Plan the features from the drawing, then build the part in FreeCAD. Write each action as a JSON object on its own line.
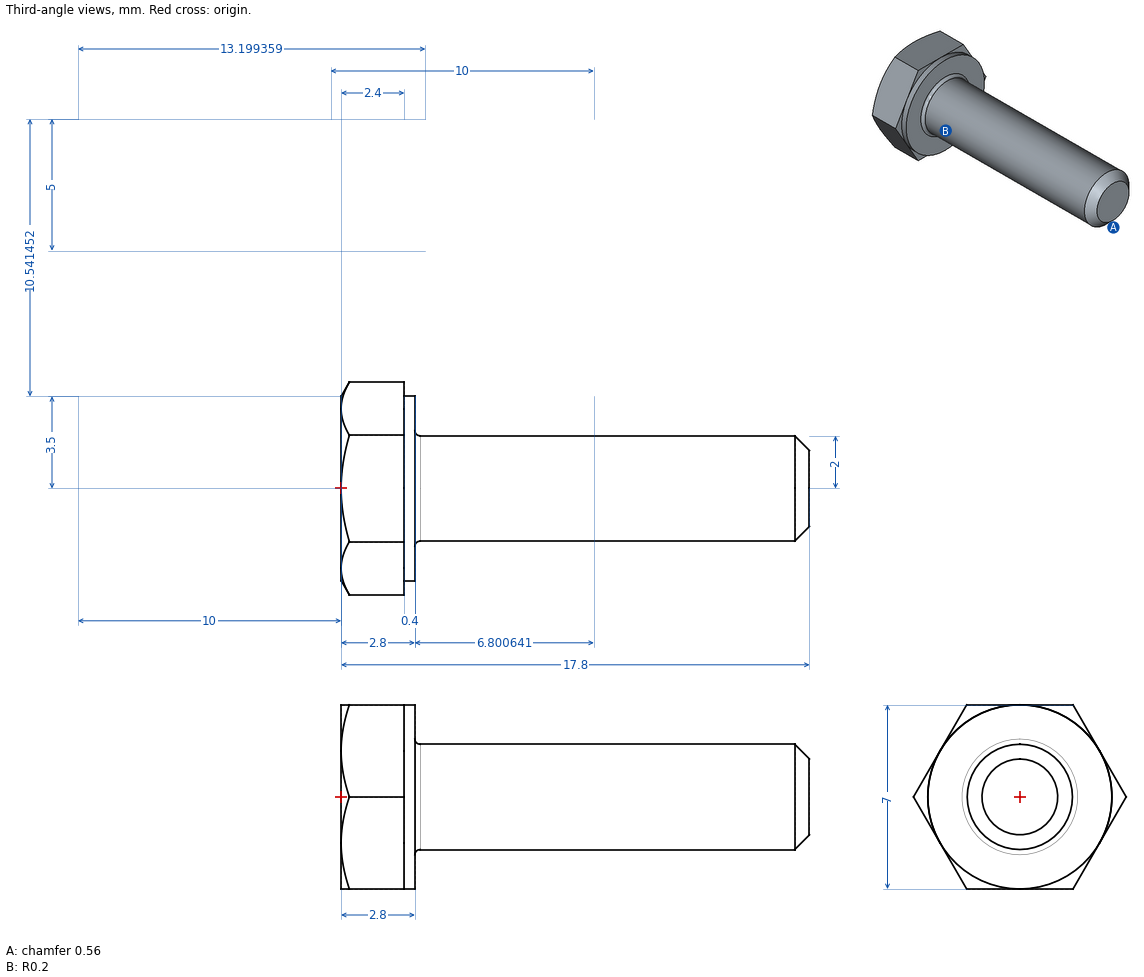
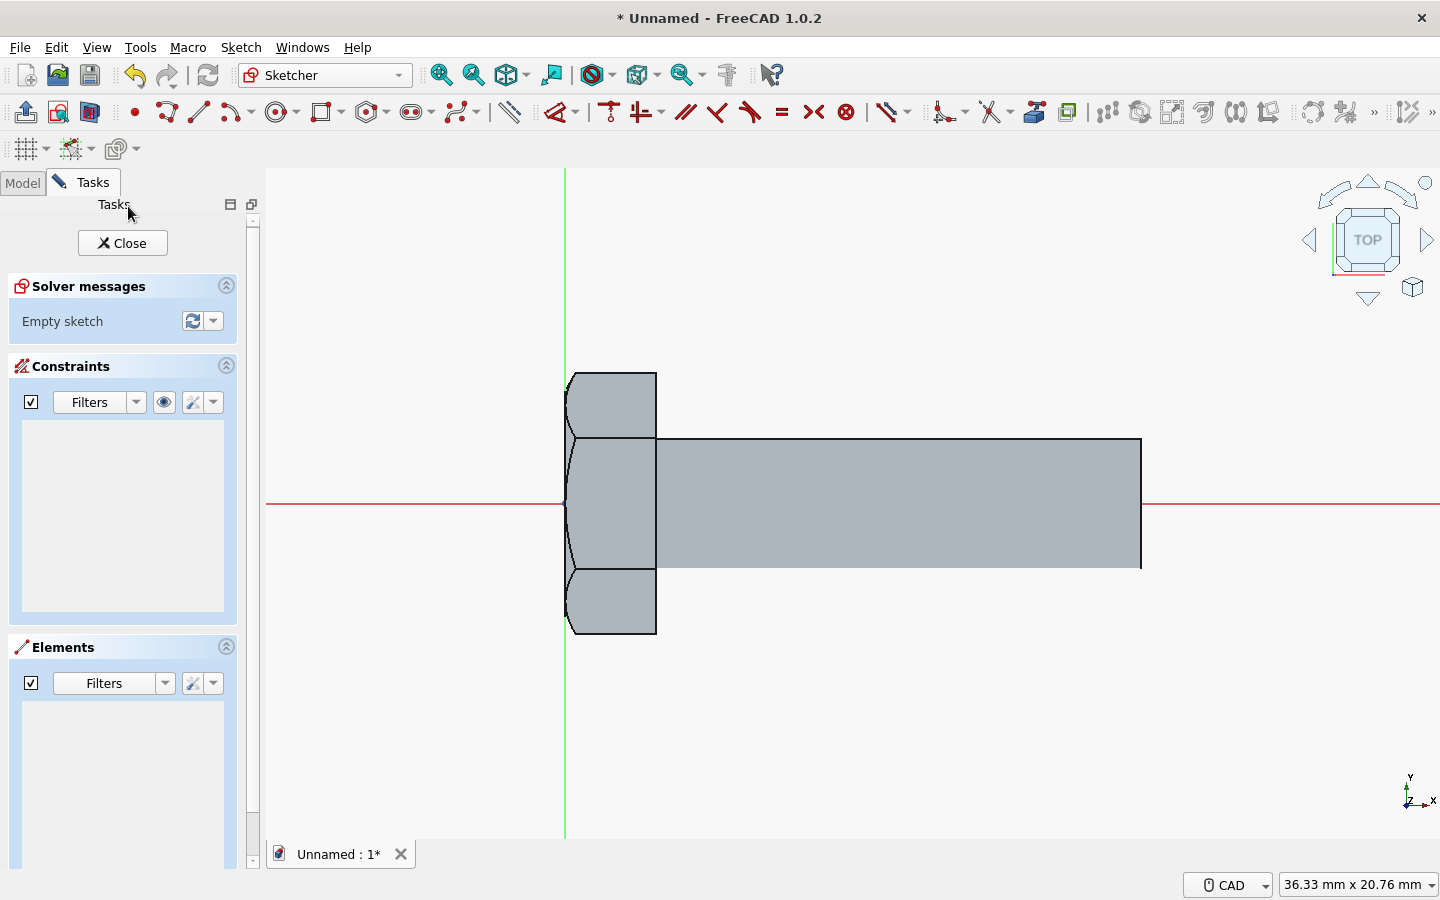
{"action": "left_click", "coordinate": [90, 112]}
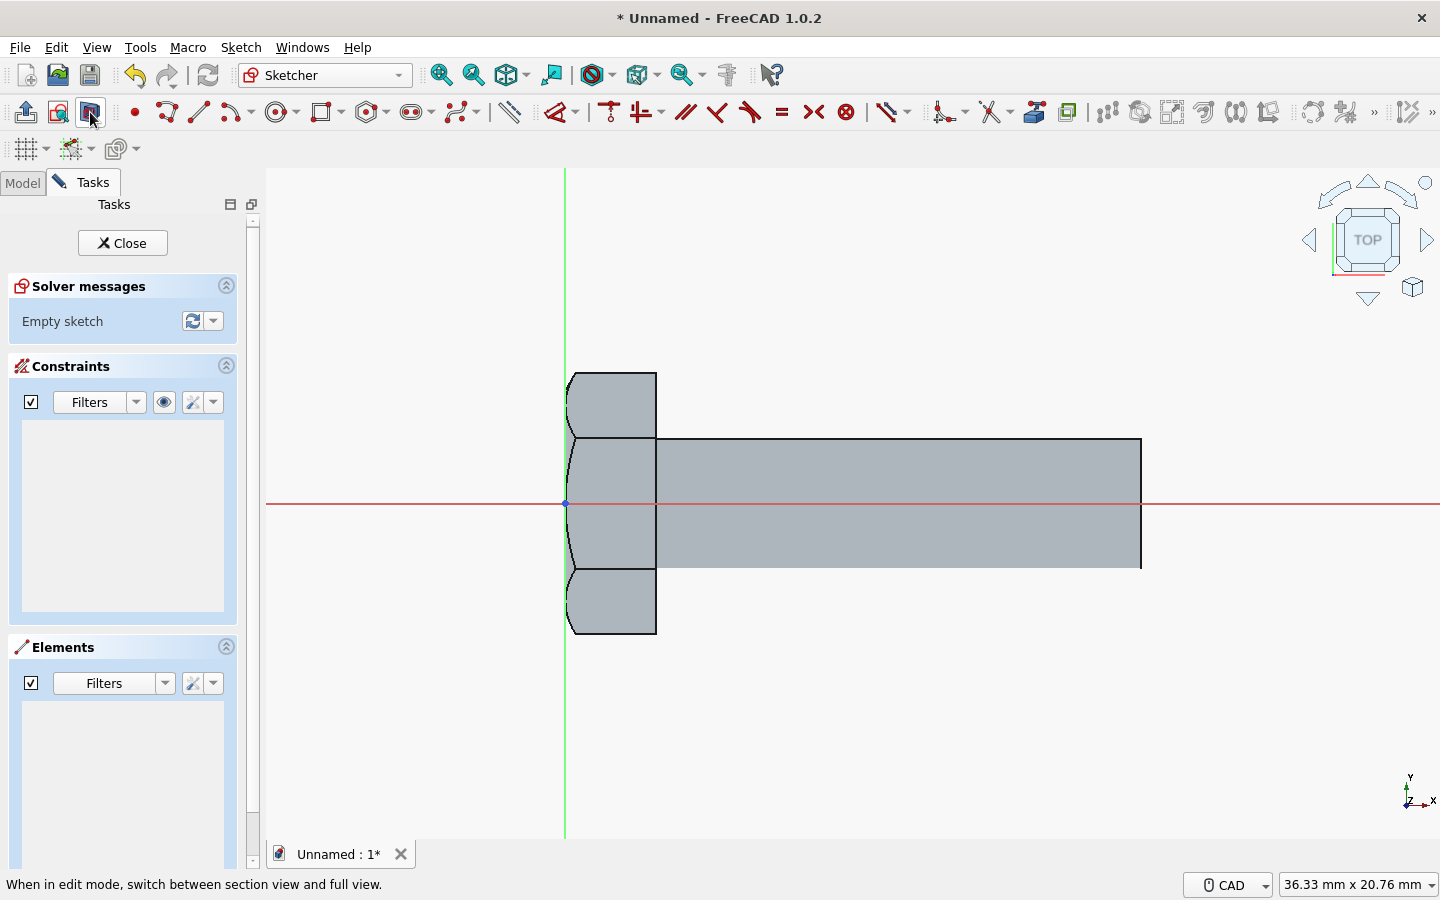
{"action": "scroll", "coordinate": [928, 811], "scroll_direction": "down", "scroll_amount": 2}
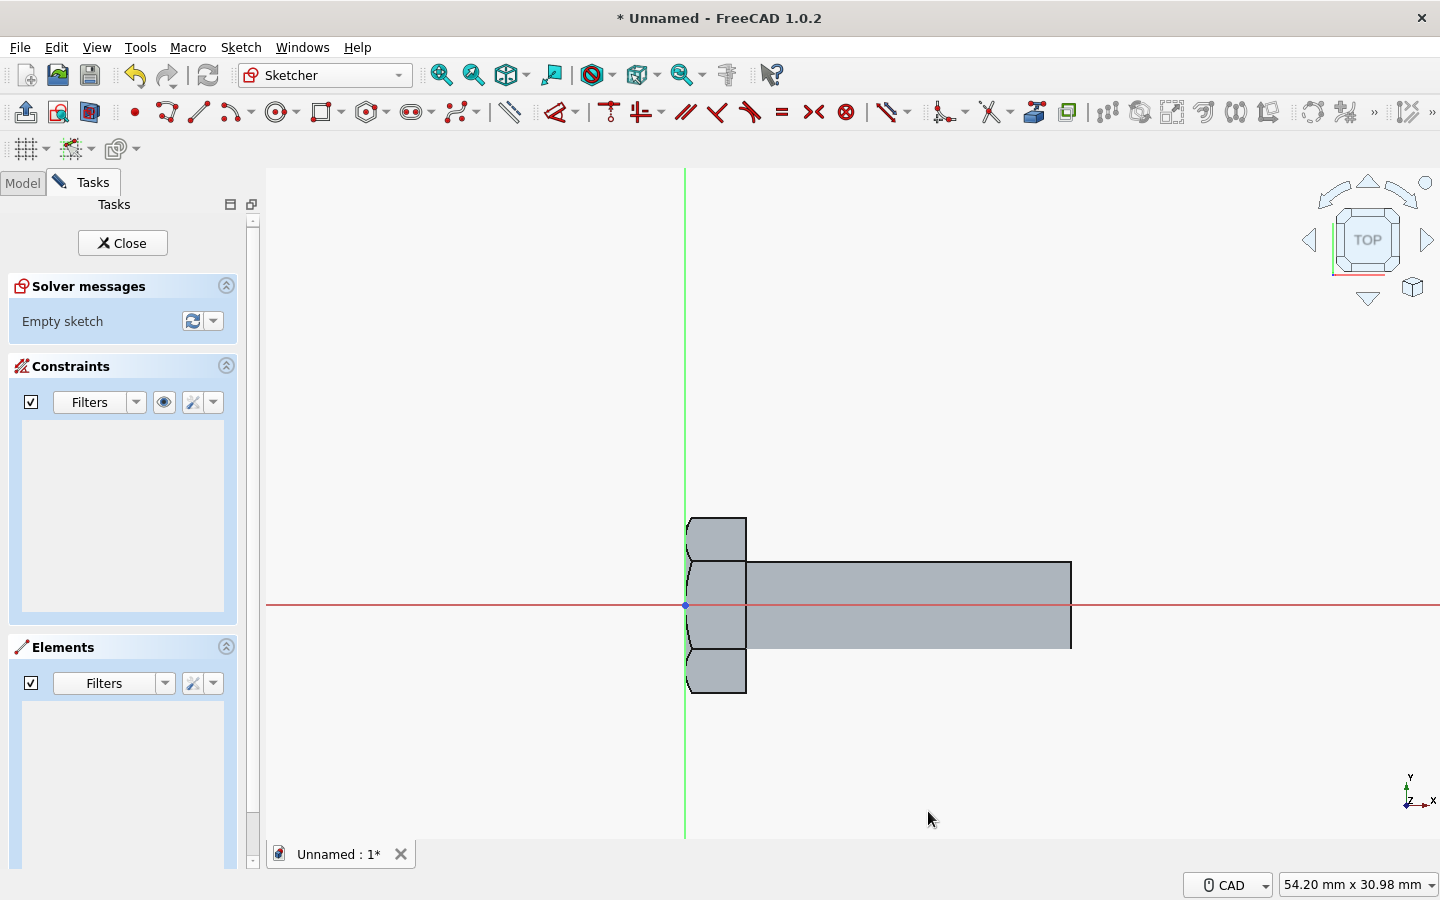
{"action": "scroll", "coordinate": [785, 351], "scroll_direction": "up", "scroll_amount": 2}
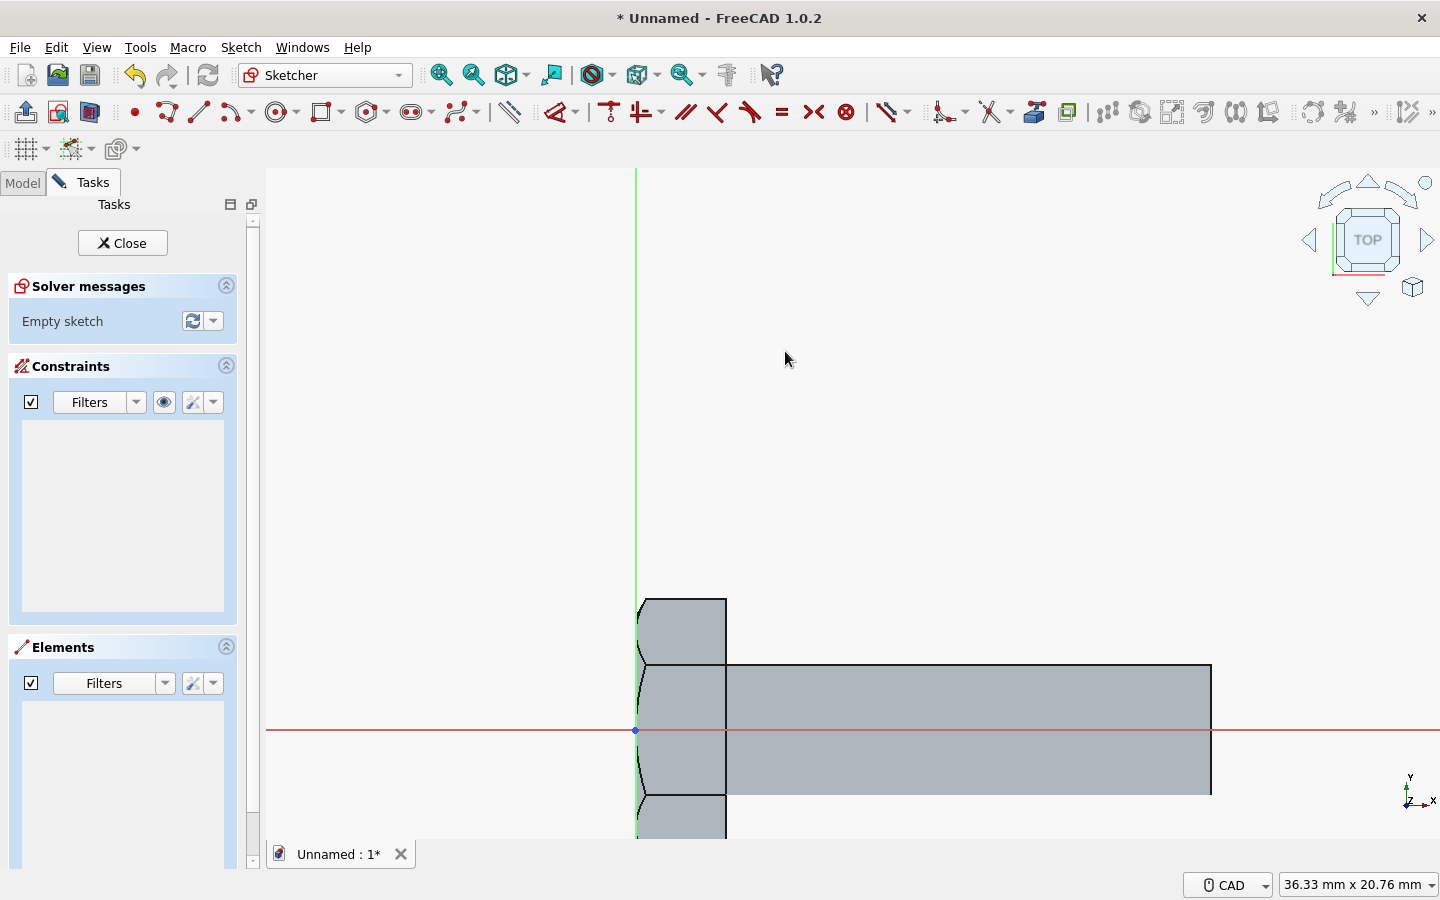
{"action": "key", "text": "g m"}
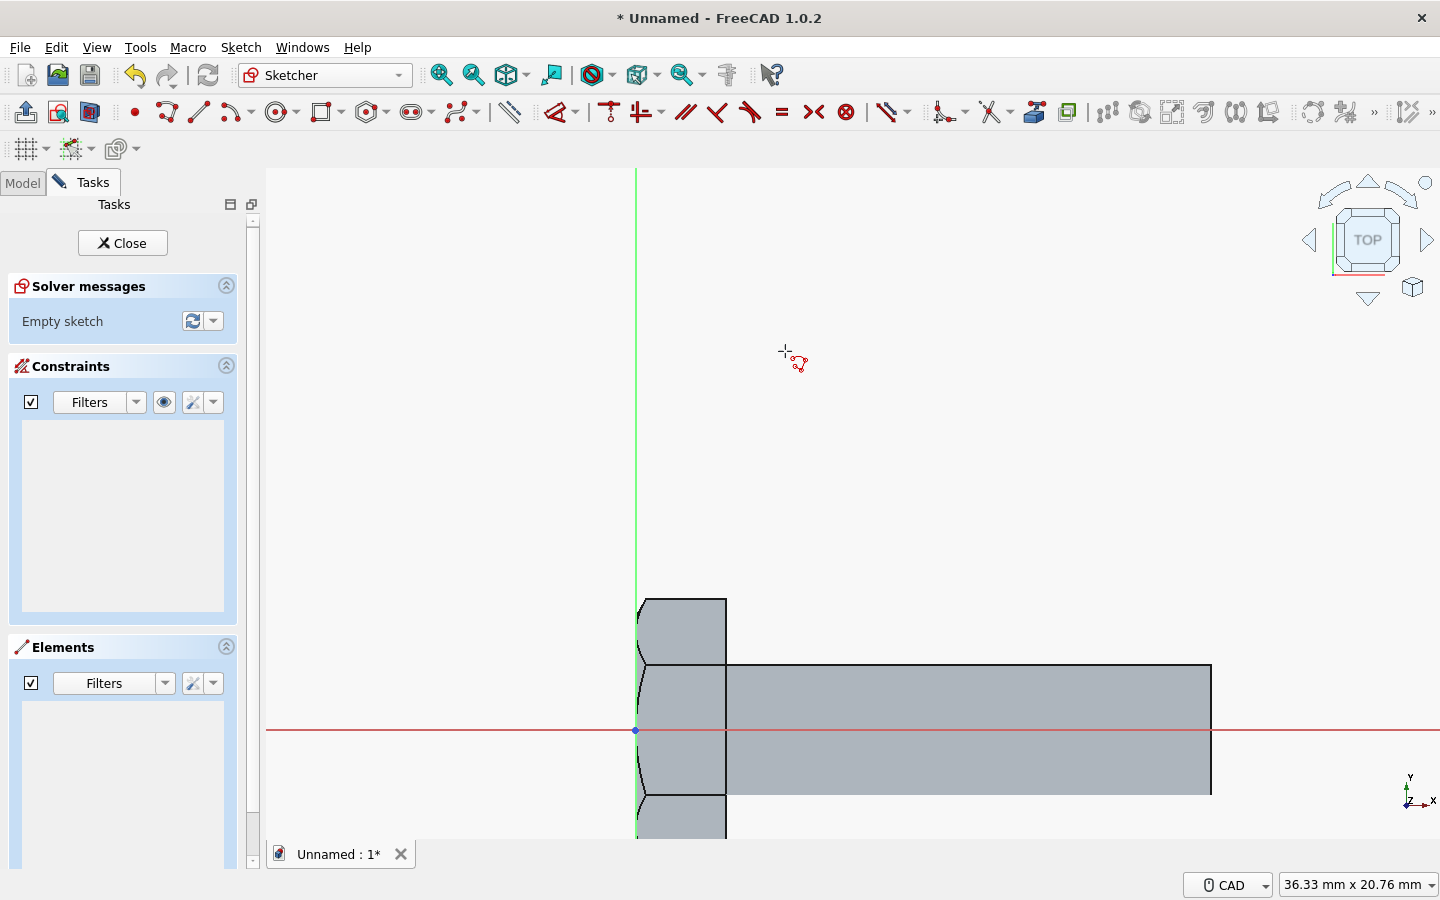
{"action": "left_click", "coordinate": [726, 617]}
{"action": "left_click", "coordinate": [946, 617]}
{"action": "left_click", "coordinate": [946, 276]}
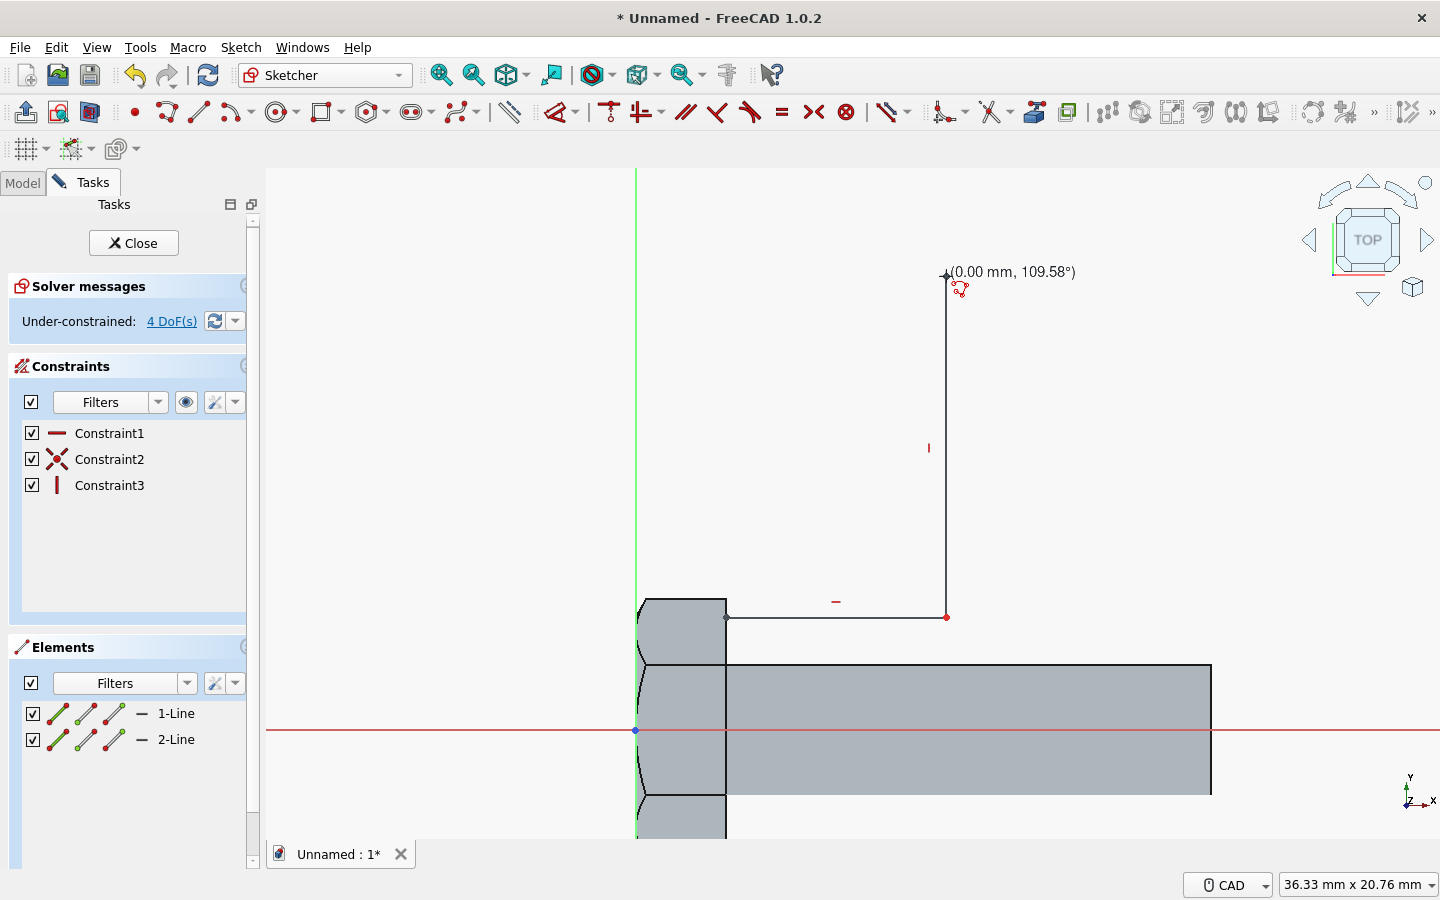
{"action": "scroll", "coordinate": [623, 276], "scroll_direction": "up", "scroll_amount": 2}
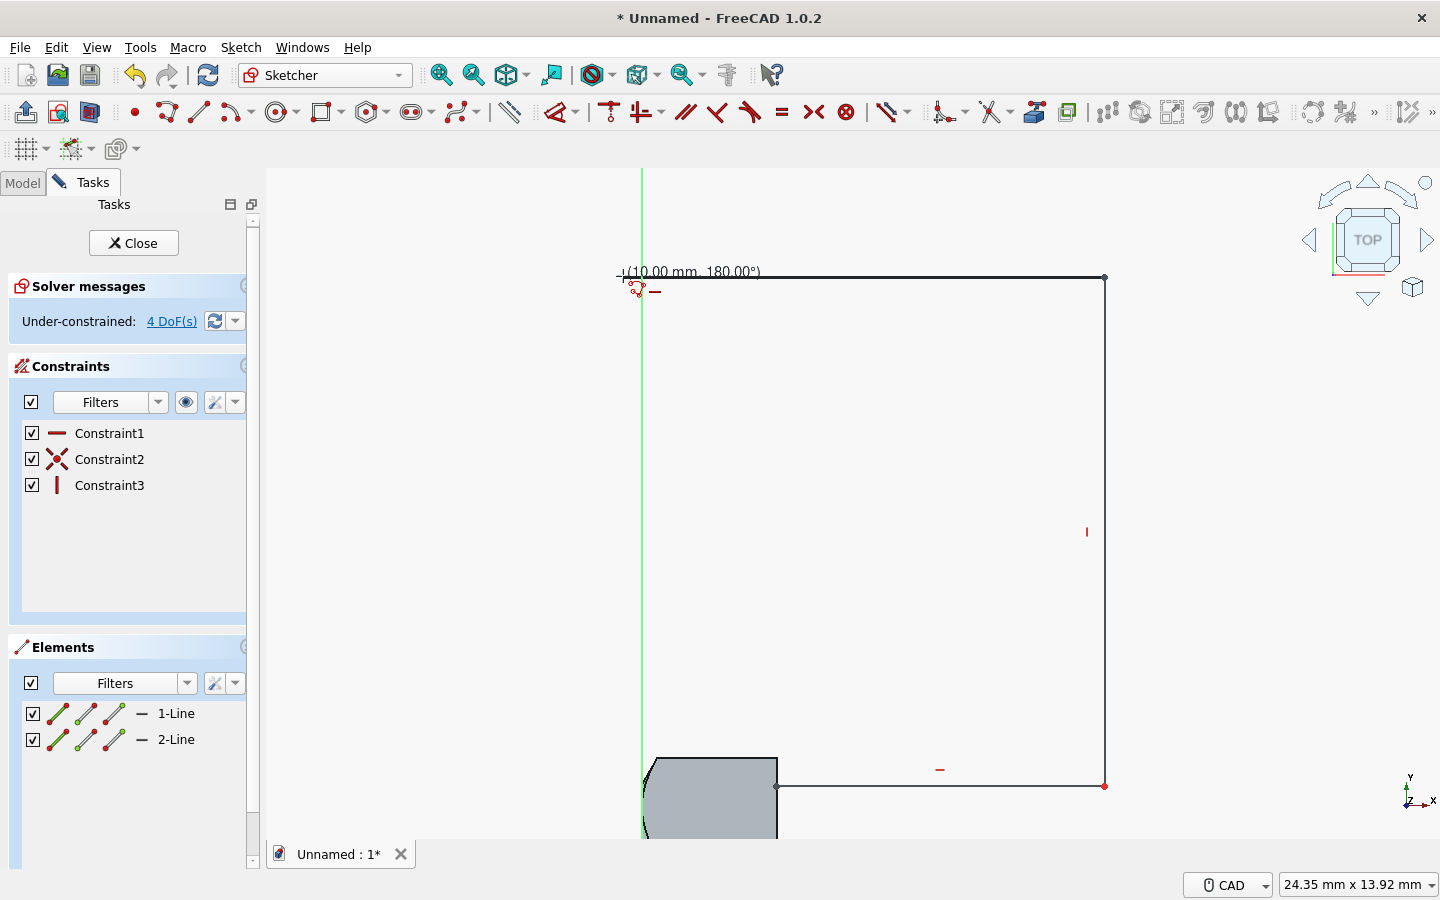
{"action": "left_click", "coordinate": [623, 276]}
{"action": "left_click", "coordinate": [623, 517]}
{"action": "left_click", "coordinate": [777, 786]}
{"action": "key", "text": "Escape"}
{"action": "key", "text": "Escape"}